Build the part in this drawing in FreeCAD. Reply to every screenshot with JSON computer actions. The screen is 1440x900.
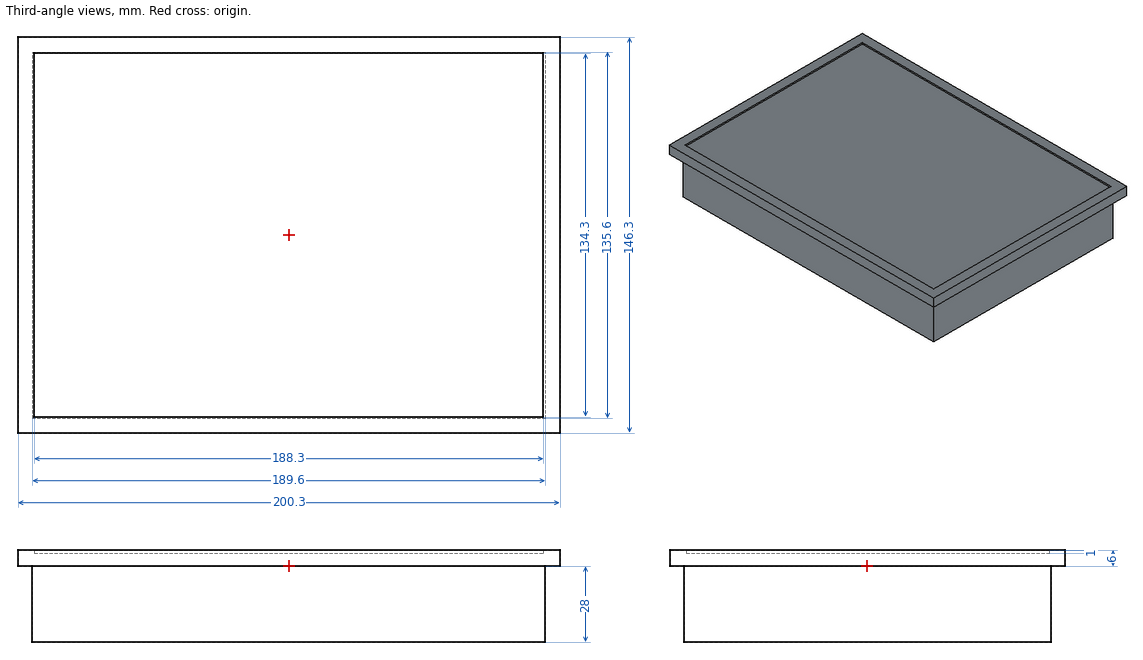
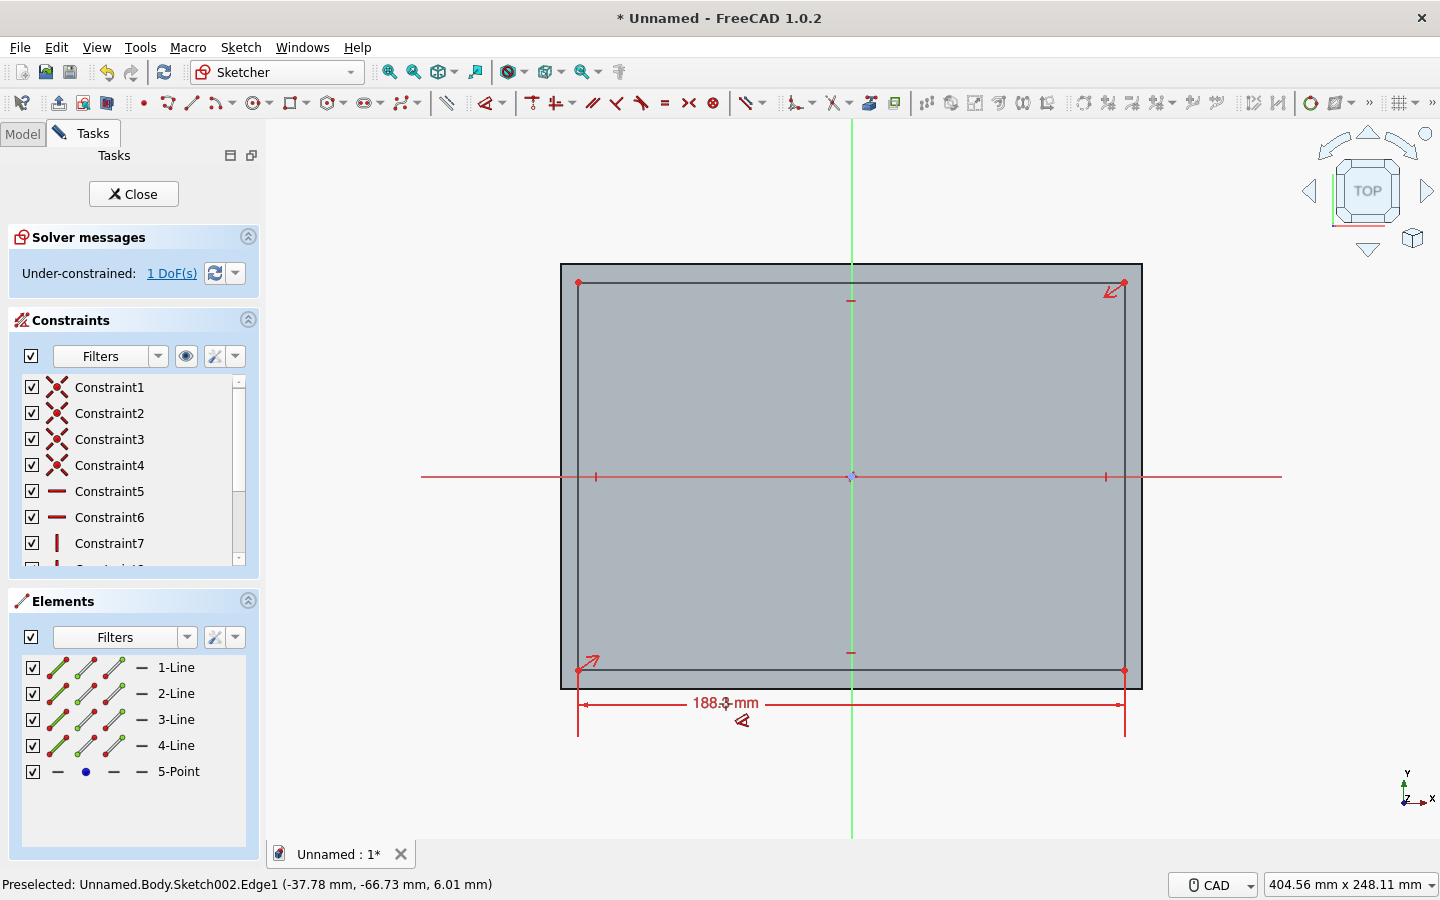
{"action": "left_click", "coordinate": [1125, 554]}
{"action": "left_click", "coordinate": [1159, 388]}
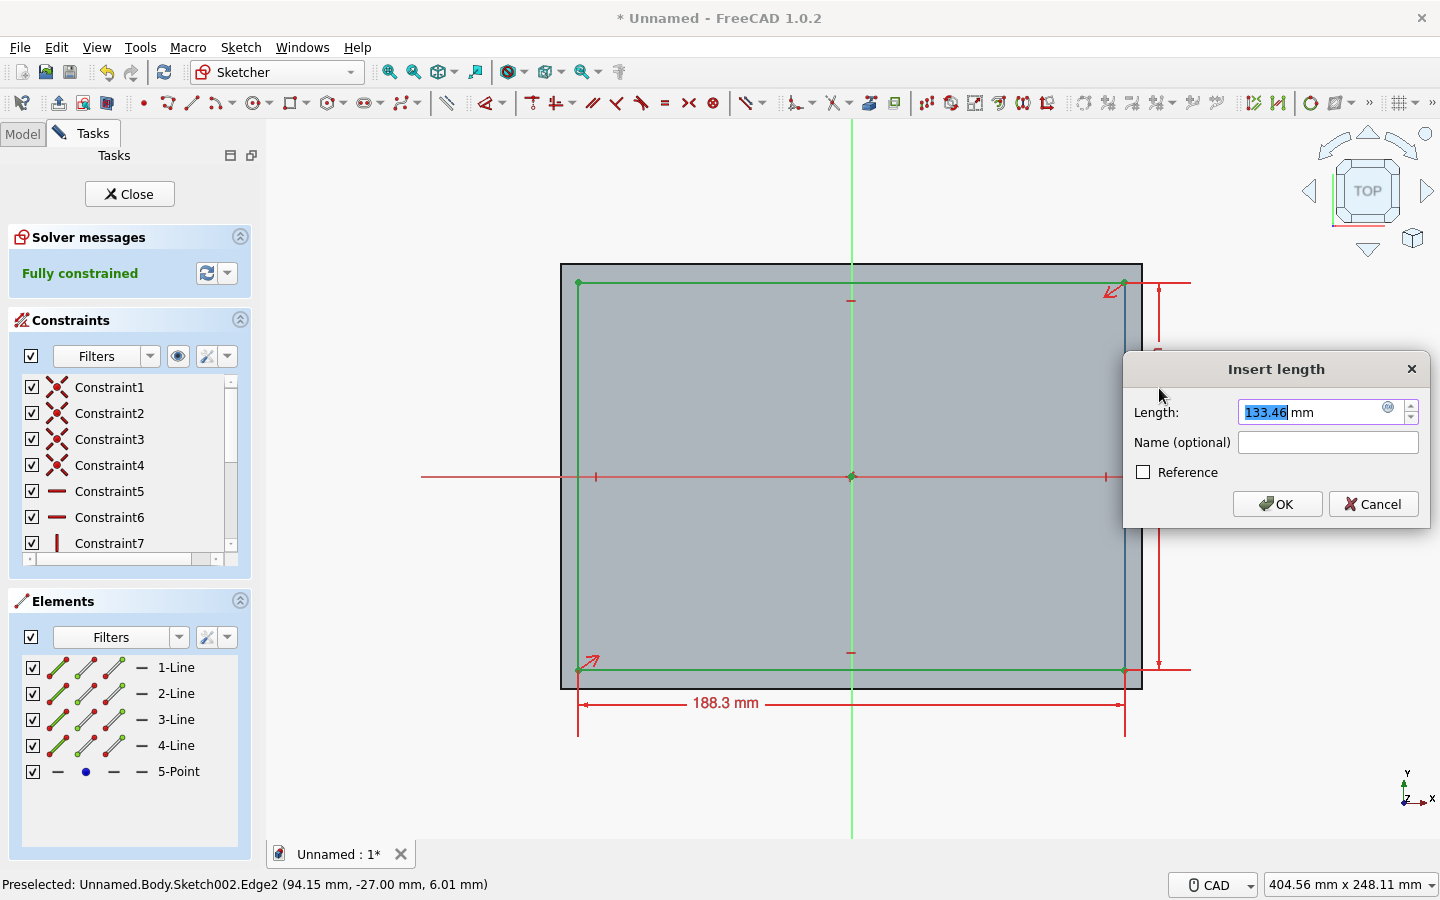
{"action": "type", "text": "134.3"}
{"action": "key", "text": "Return"}
{"action": "key", "text": "Escape"}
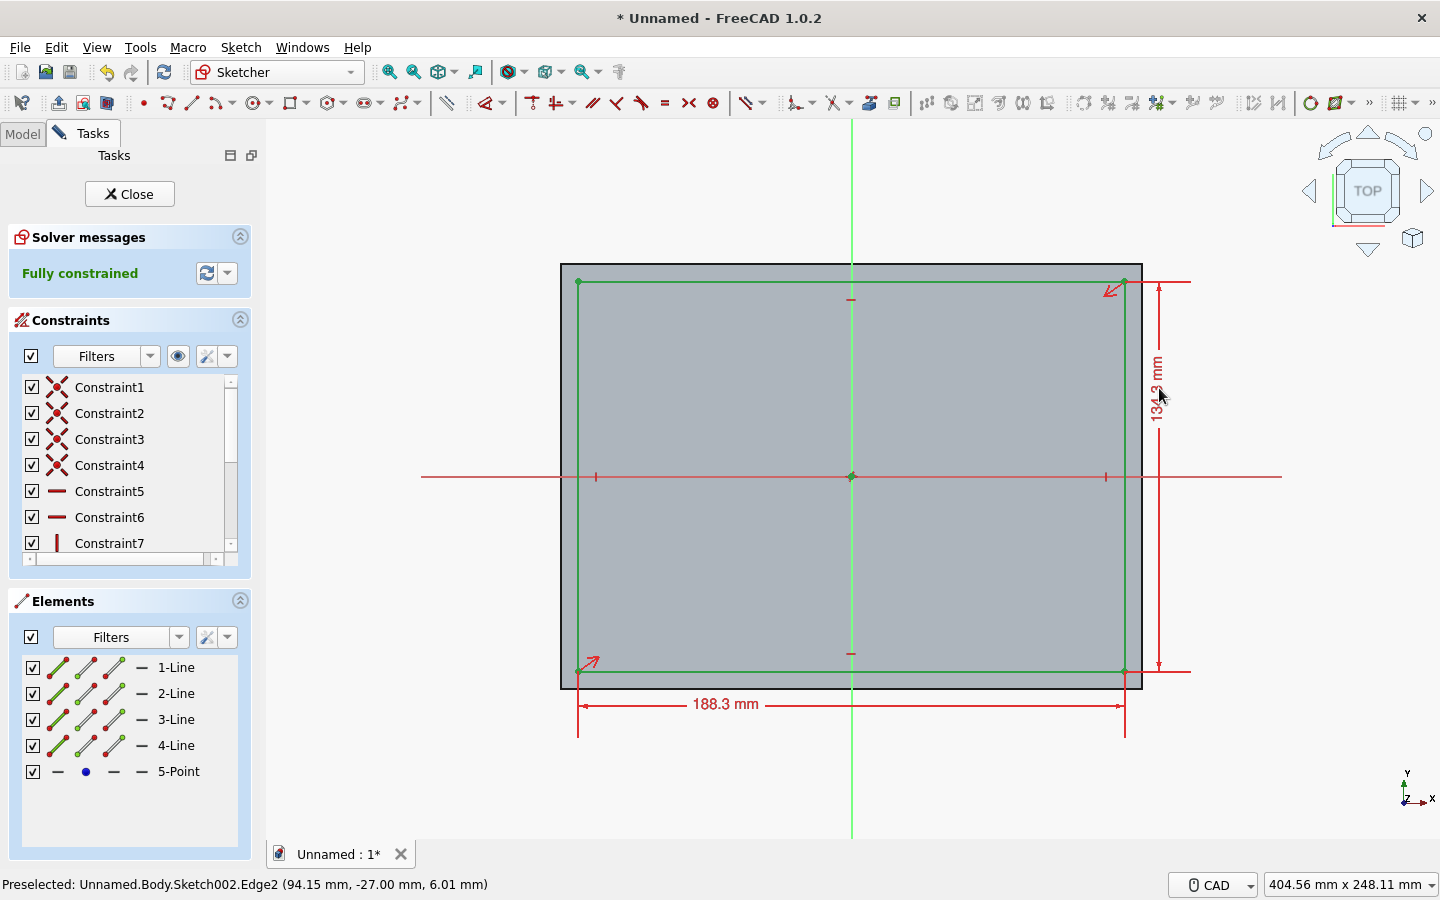
{"action": "left_click", "coordinate": [130, 194]}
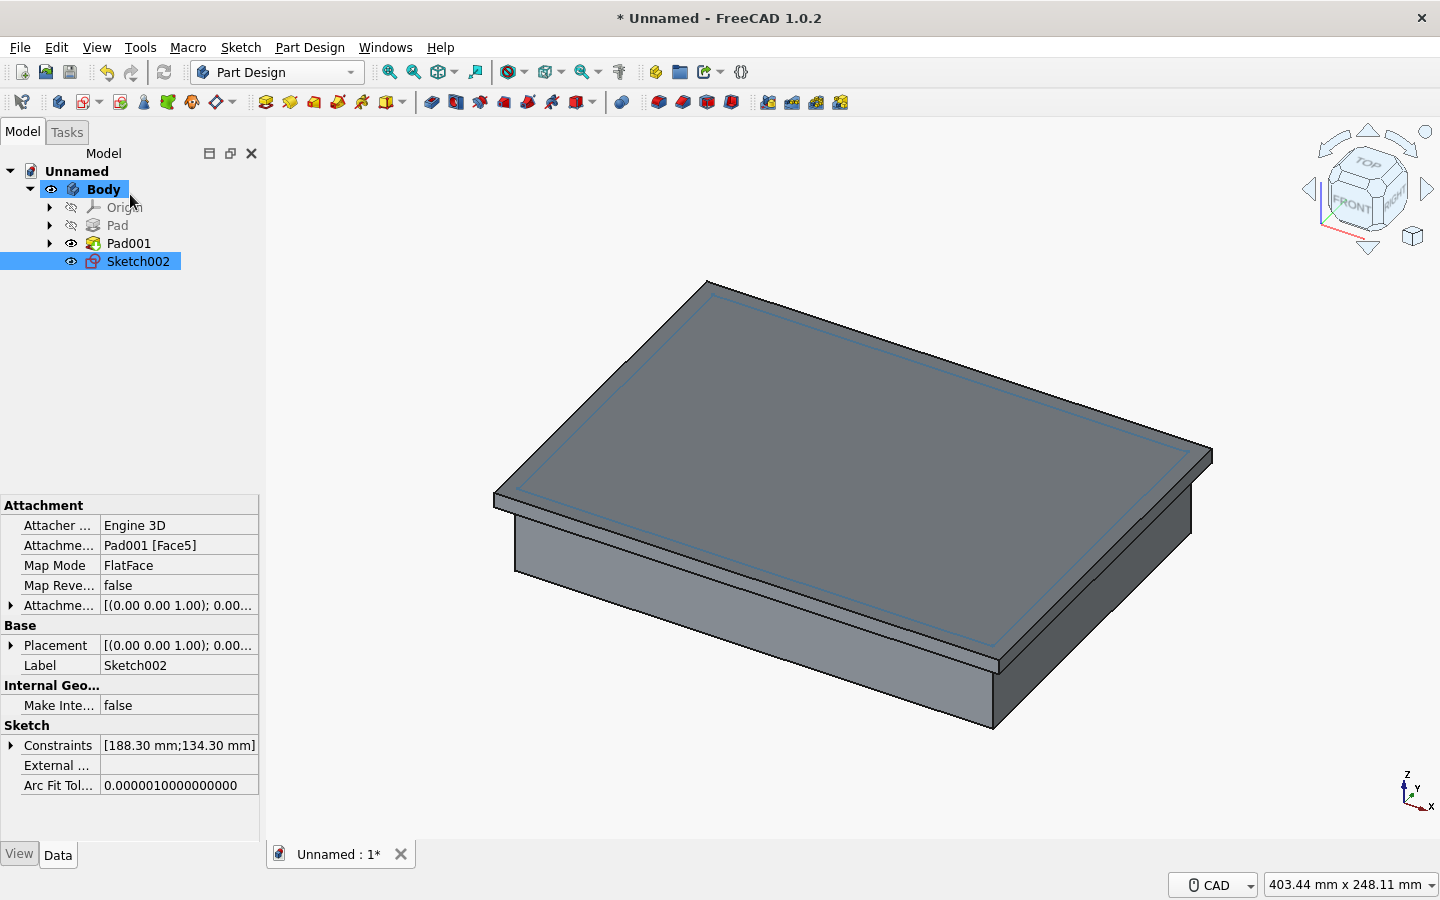
{"action": "left_click", "coordinate": [432, 102]}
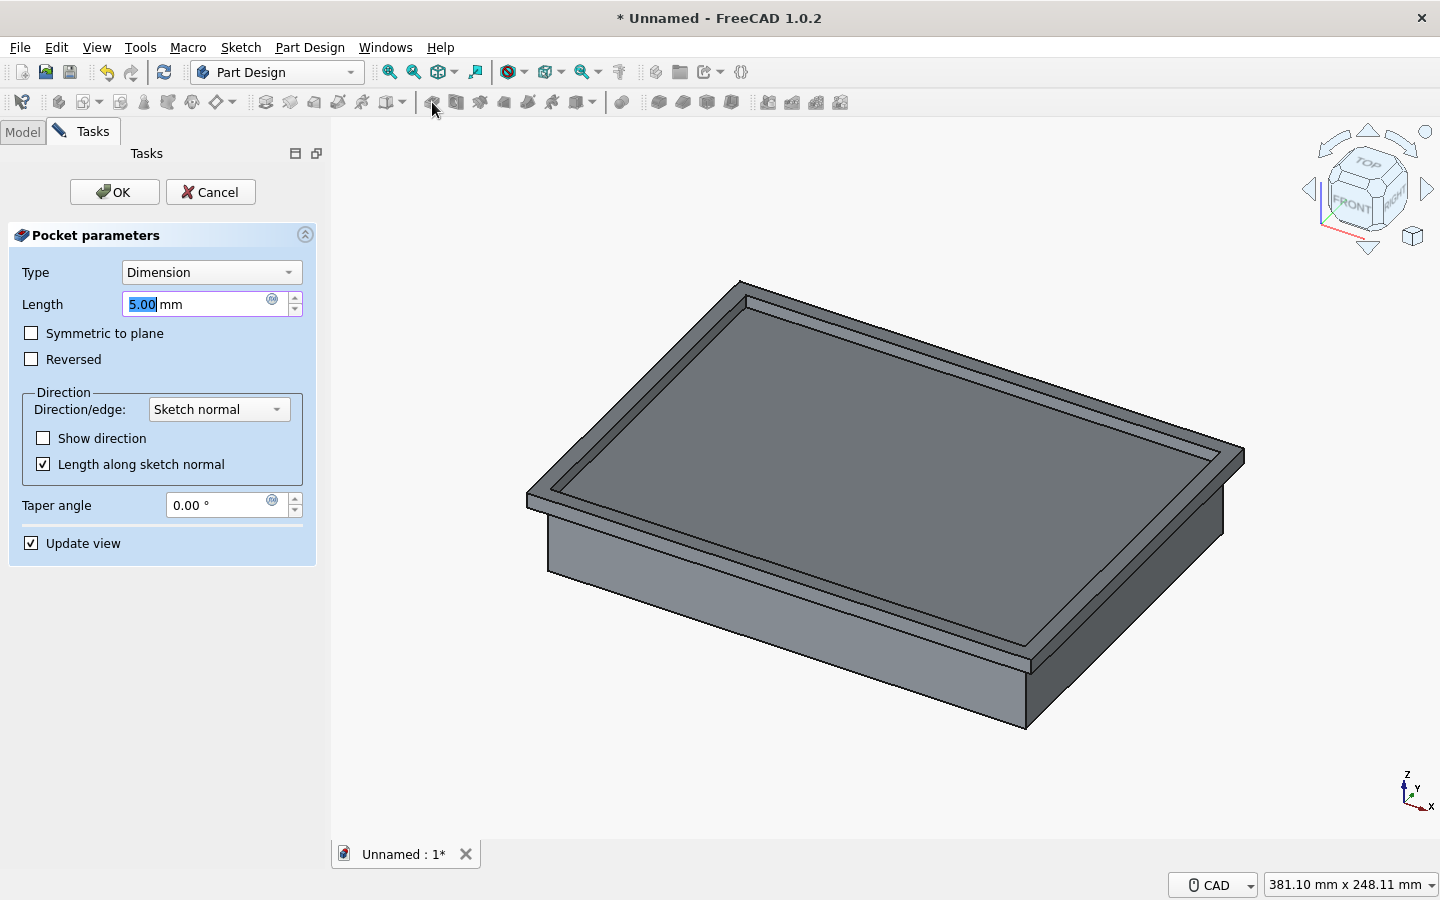
{"action": "type", "text": "1"}
{"action": "key", "text": "Tab"}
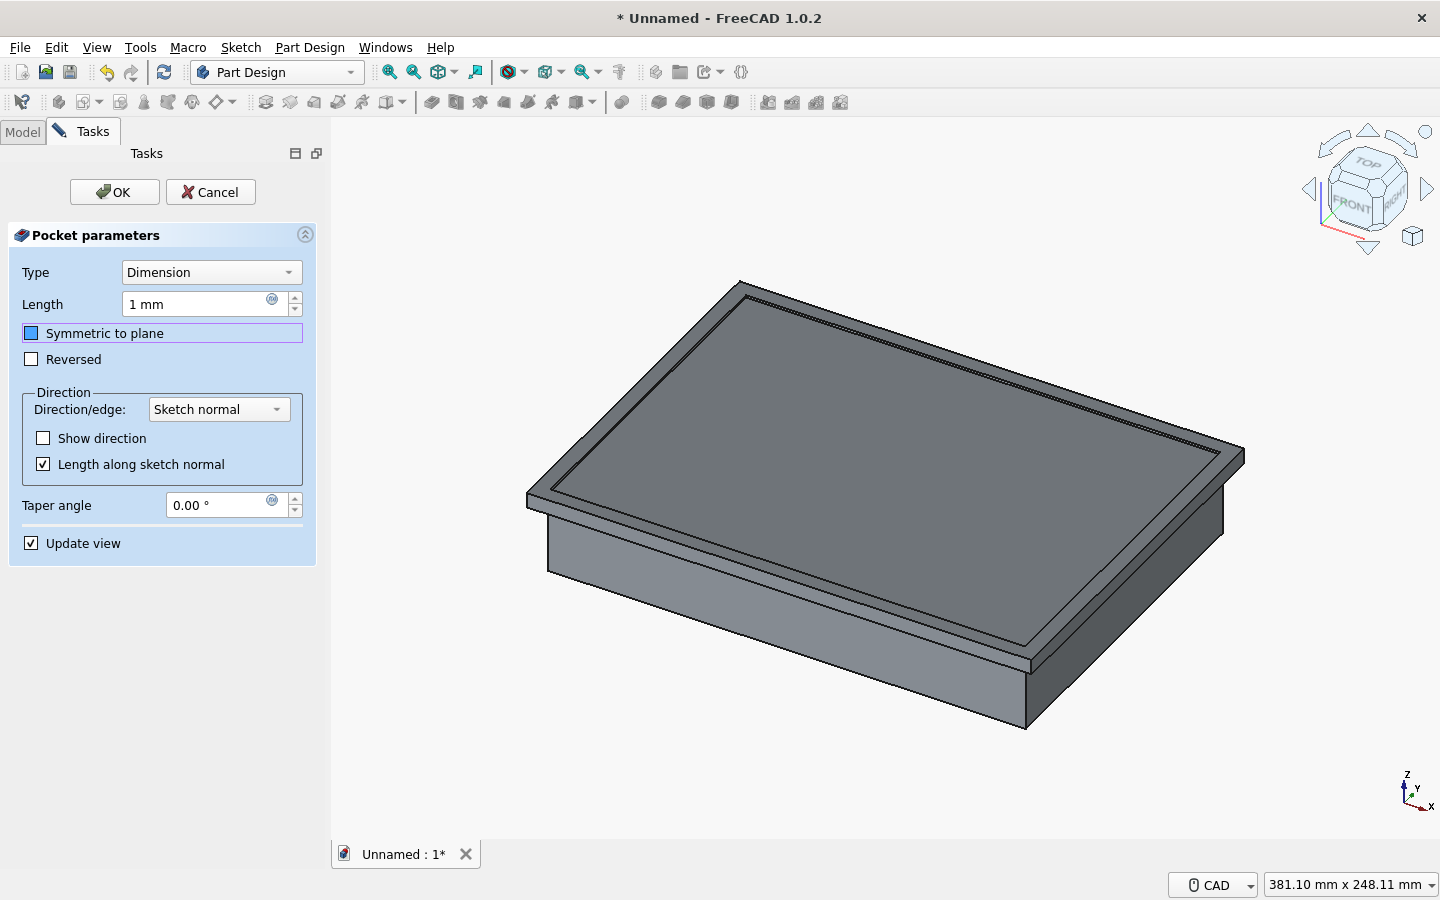
{"action": "left_click", "coordinate": [115, 192]}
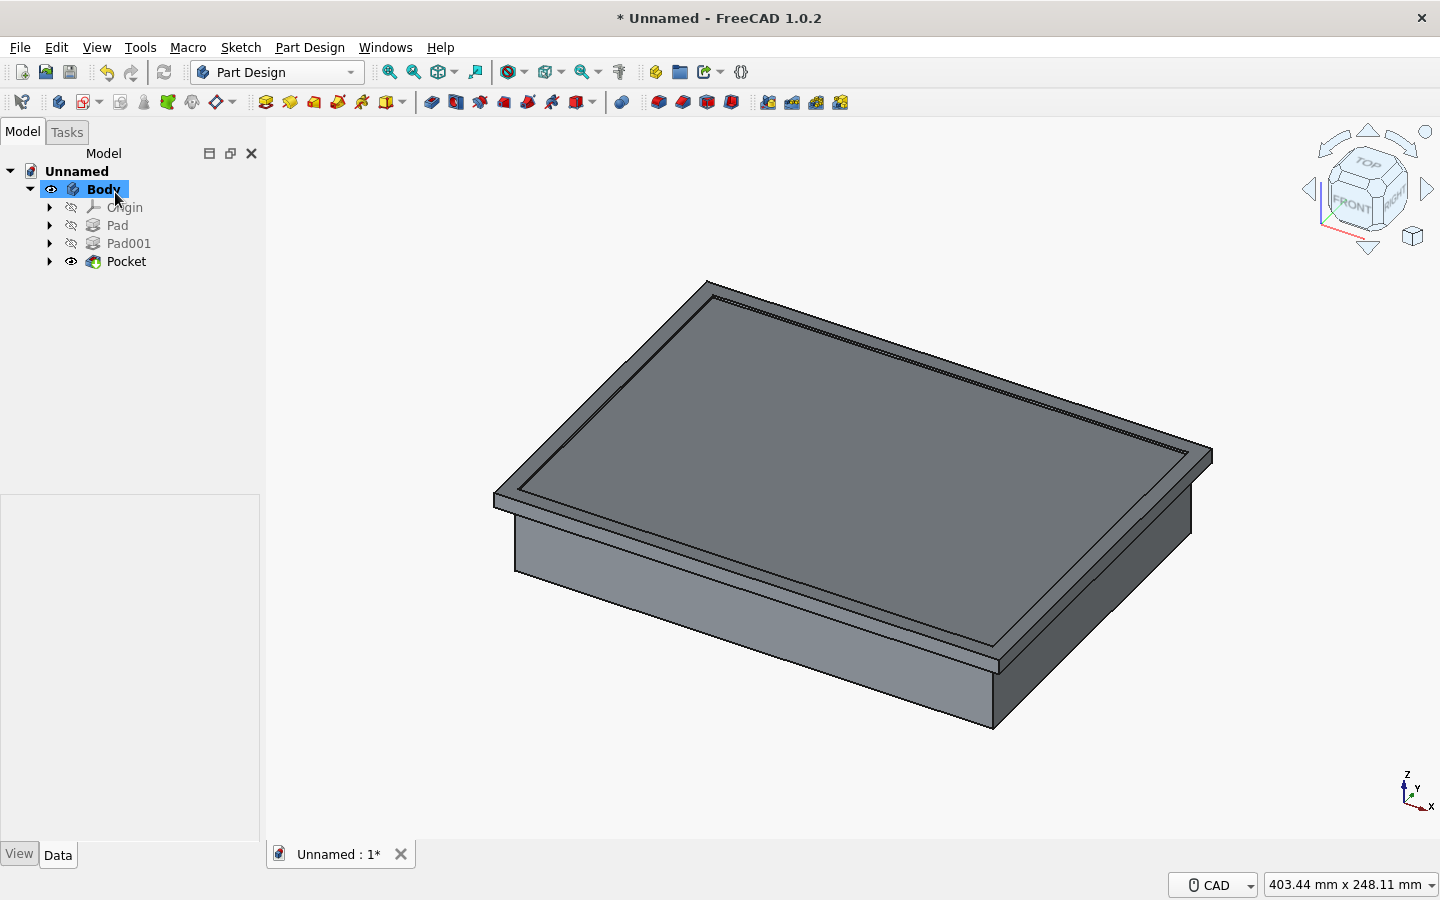
{"action": "key", "text": "0"}